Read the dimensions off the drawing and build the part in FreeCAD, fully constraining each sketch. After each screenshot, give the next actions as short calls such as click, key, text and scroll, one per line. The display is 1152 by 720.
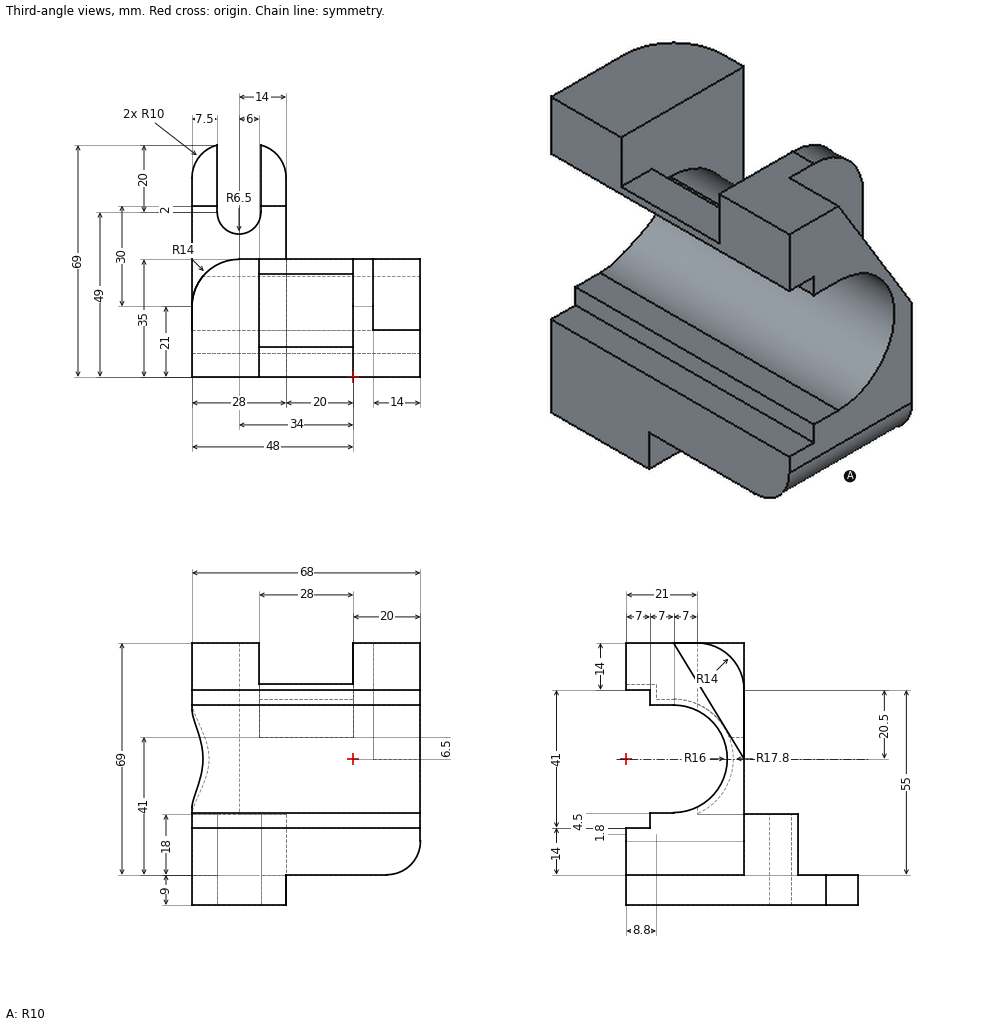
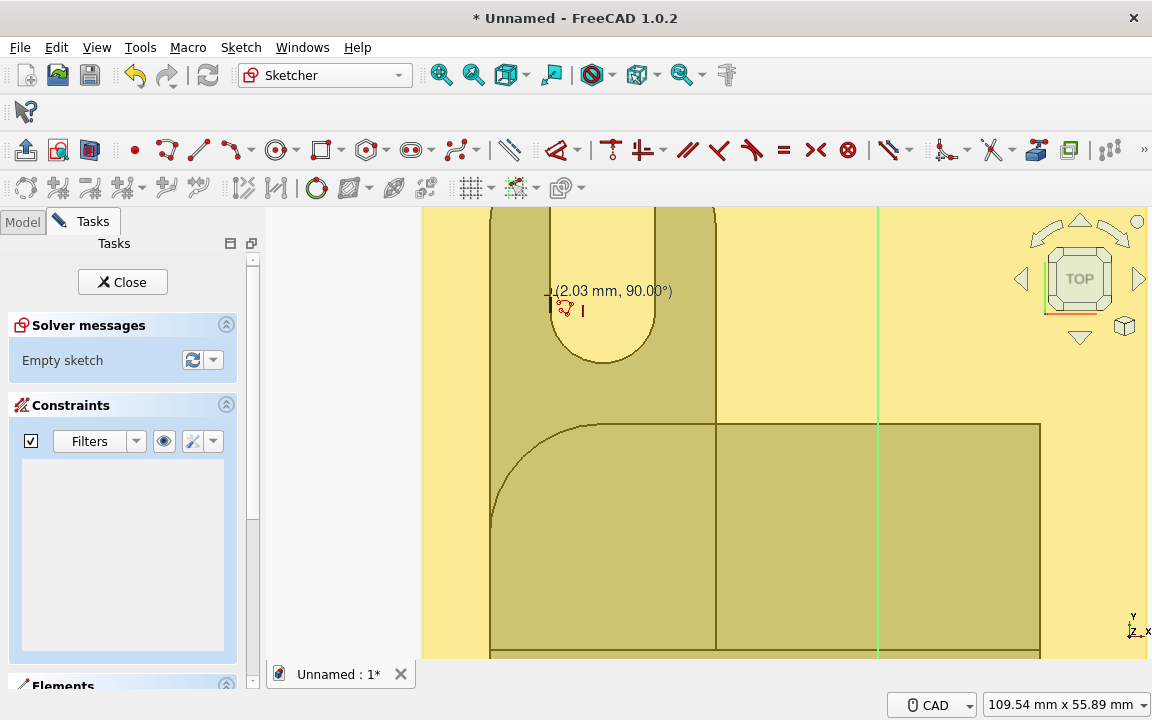
click(551, 295)
click(490, 295)
click(490, 537)
right_click(490, 537)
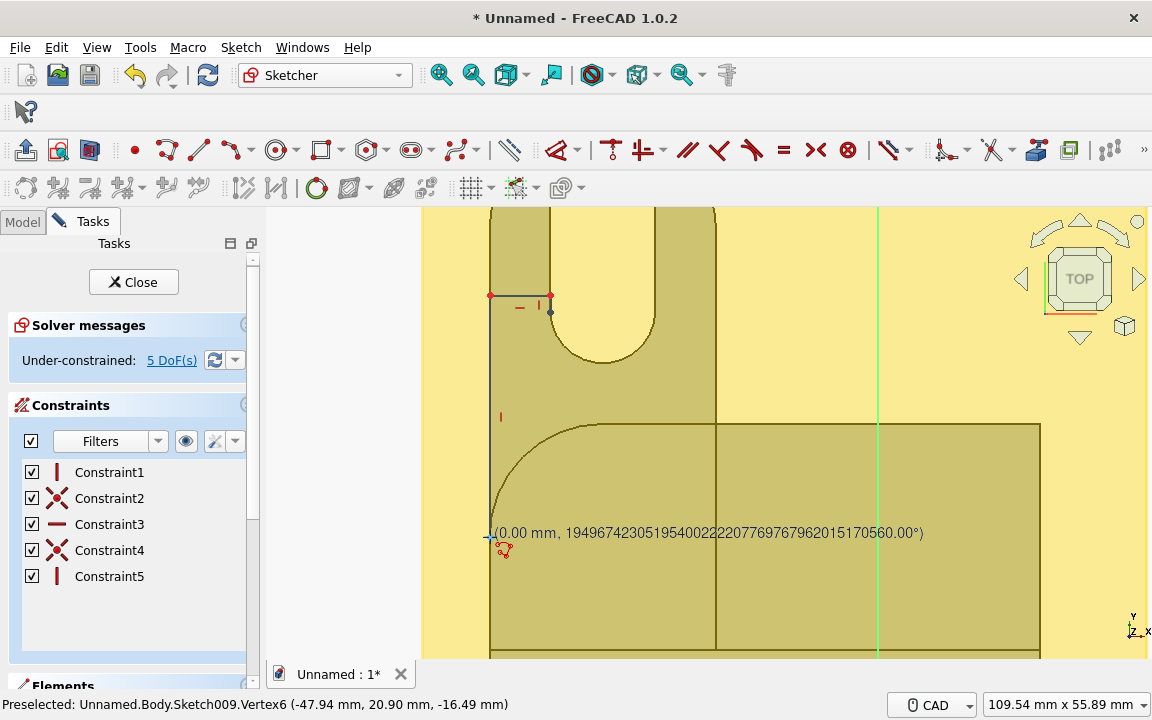
click(603, 424)
click(716, 424)
click(716, 295)
click(655, 295)
click(655, 311)
right_click(655, 311)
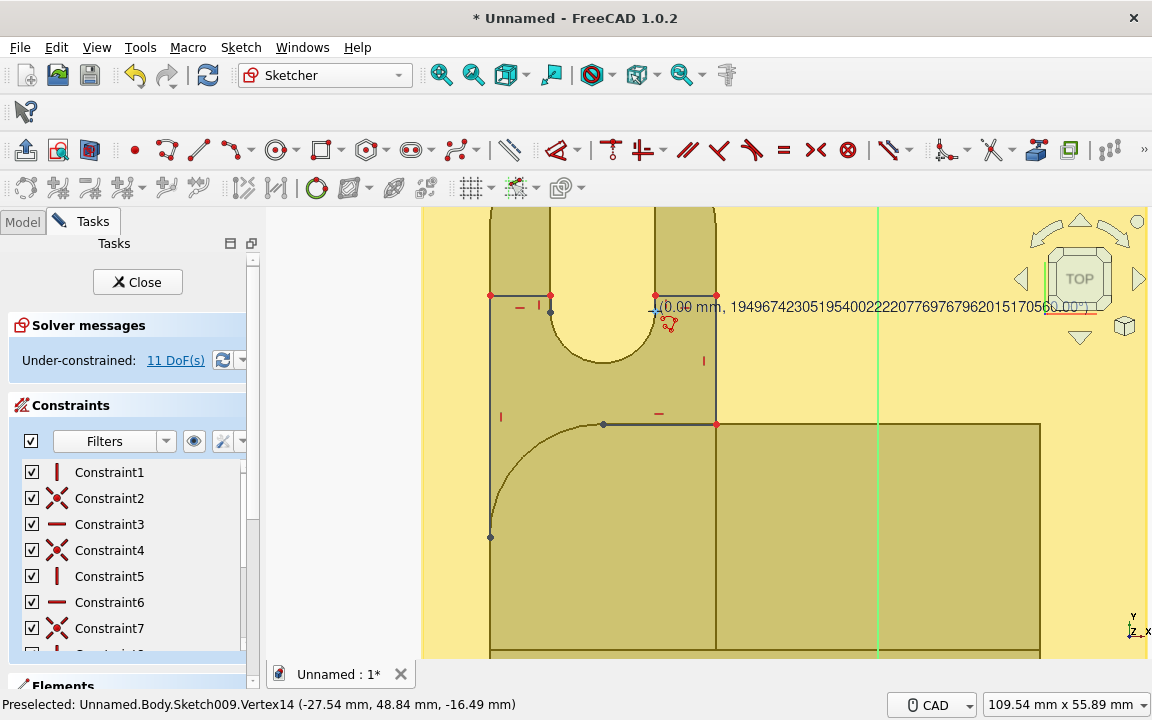
key(g)
key(3)
key(a)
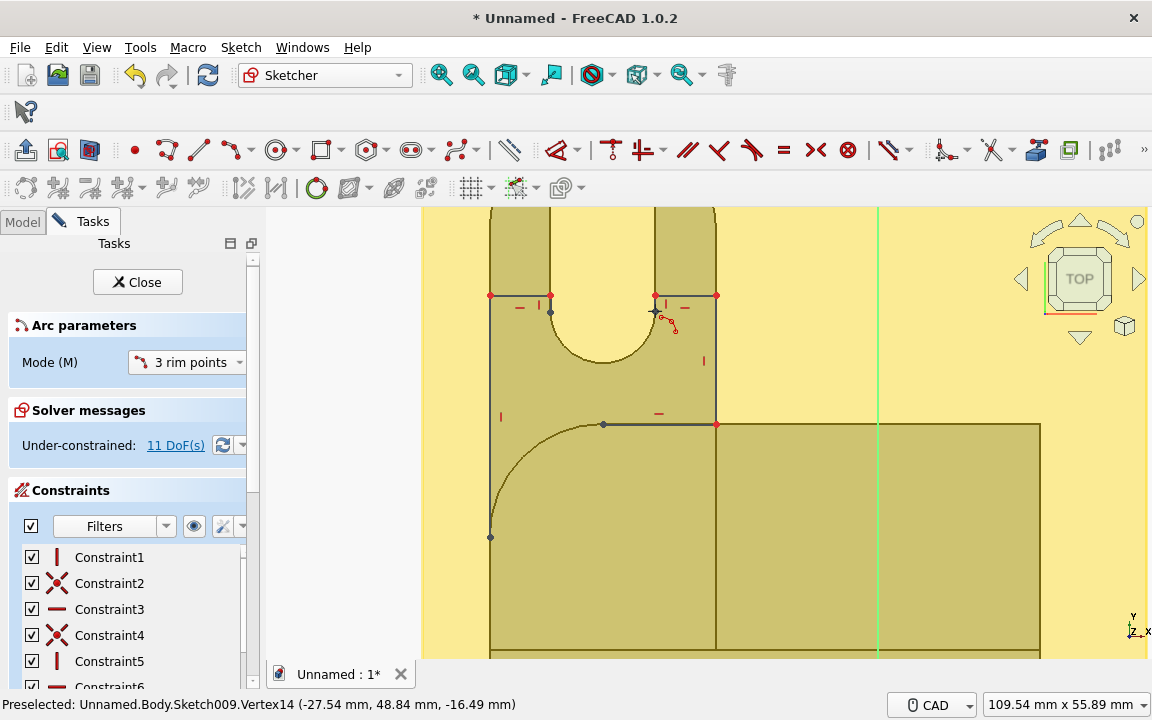
click(490, 538)
click(603, 425)
click(523, 457)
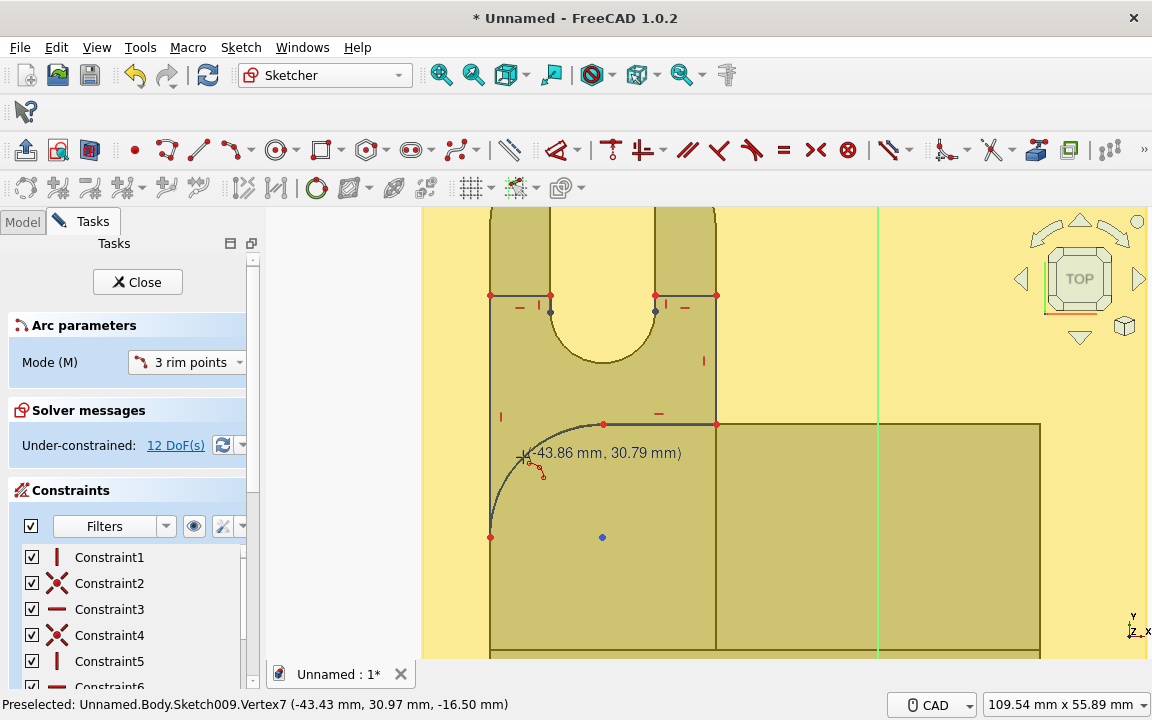
scroll(655, 311, up, 4)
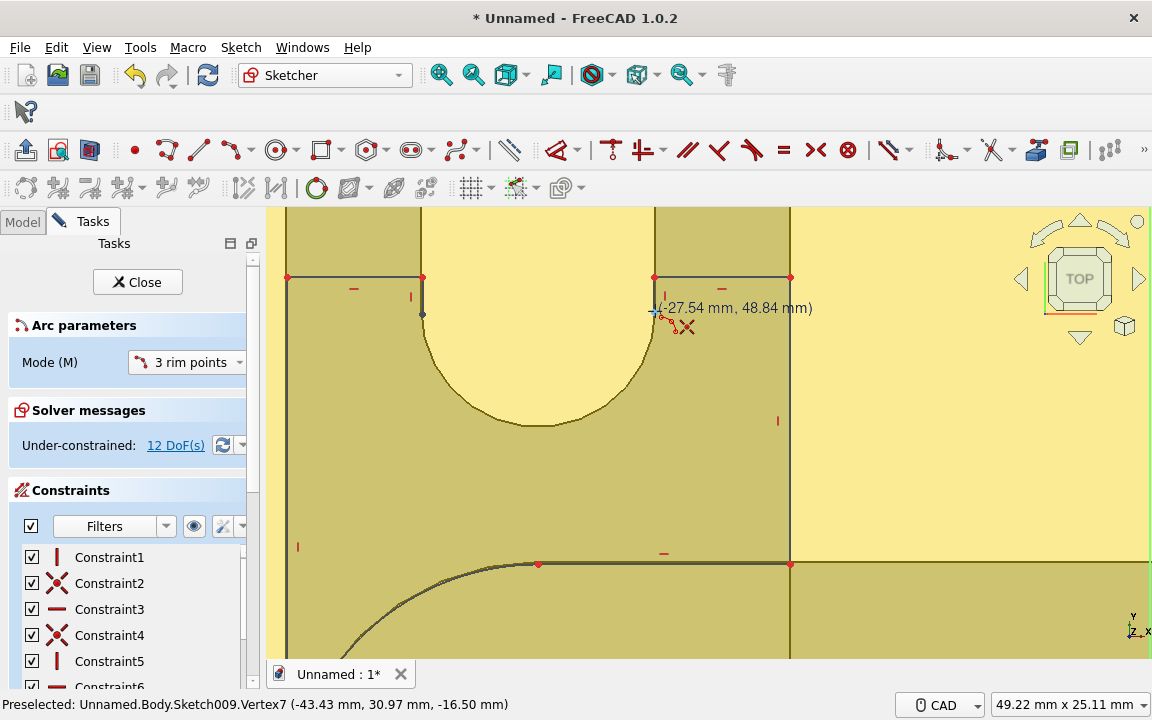
click(654, 313)
click(423, 315)
click(538, 427)
key(Escape)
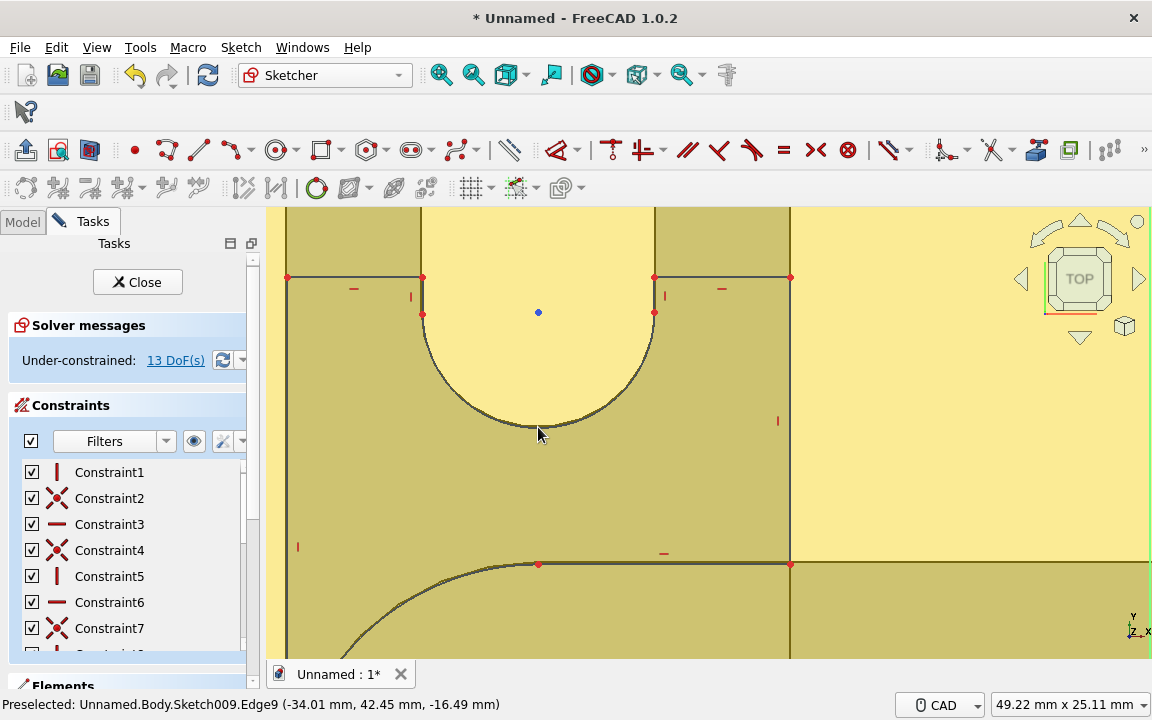
scroll(423, 304, up, 2)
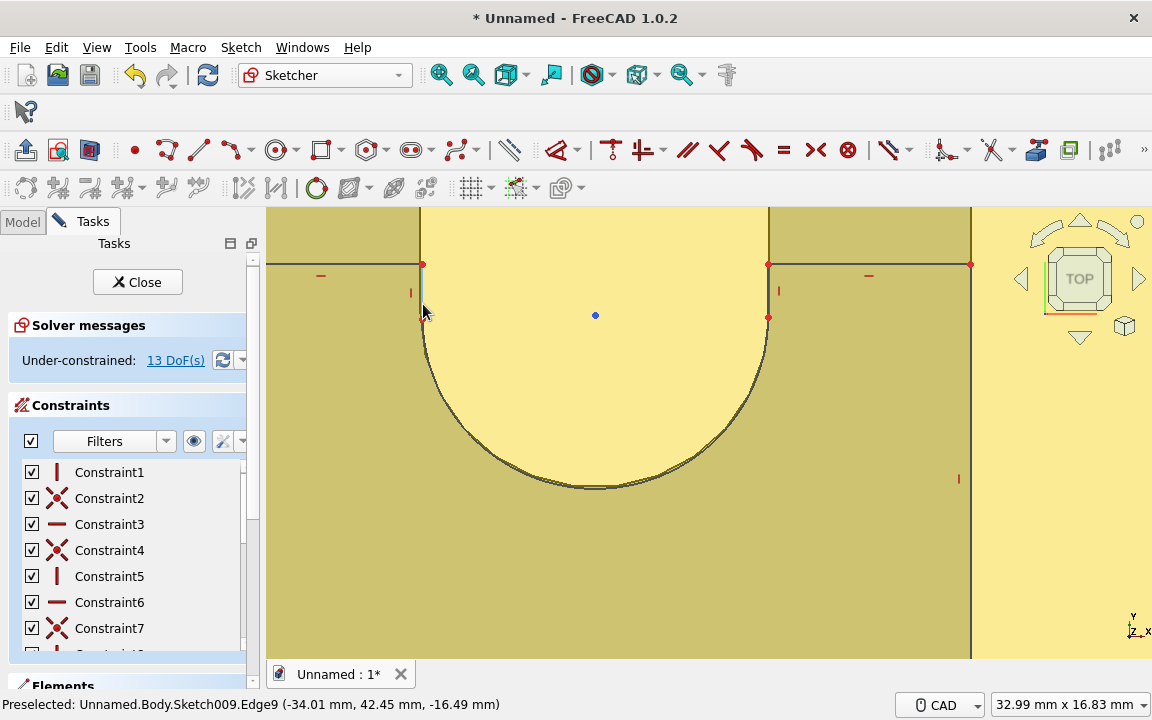
click(422, 303)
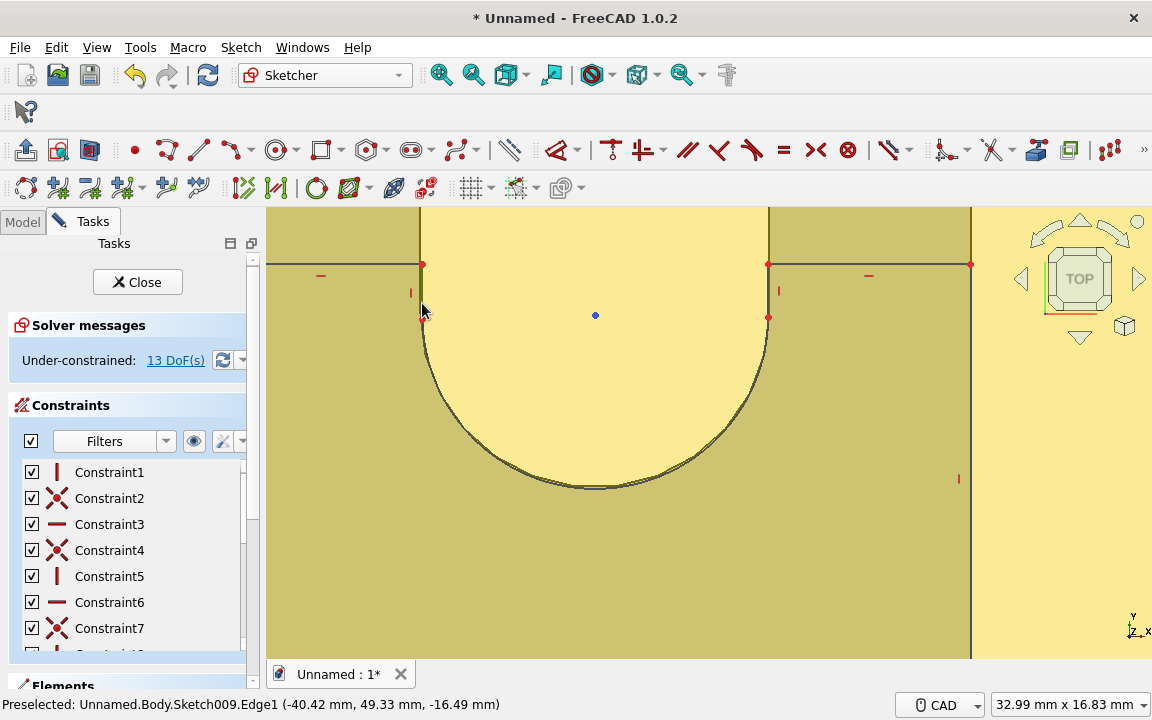
scroll(584, 304, down, 8)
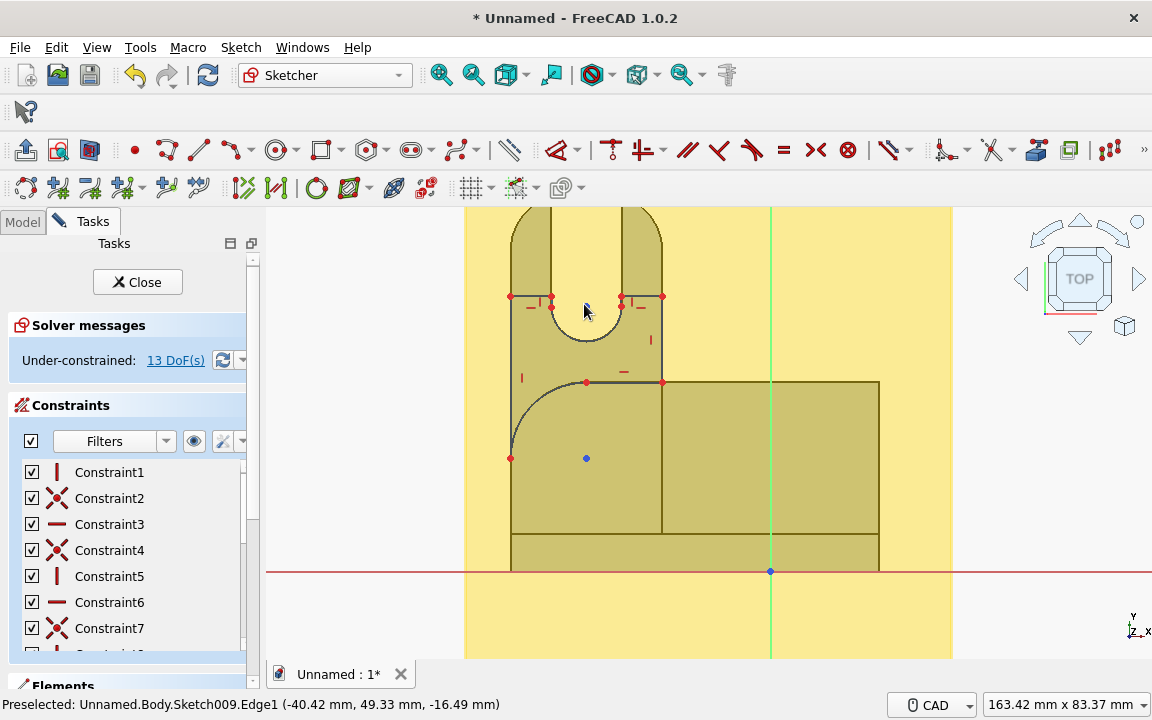
click(566, 335)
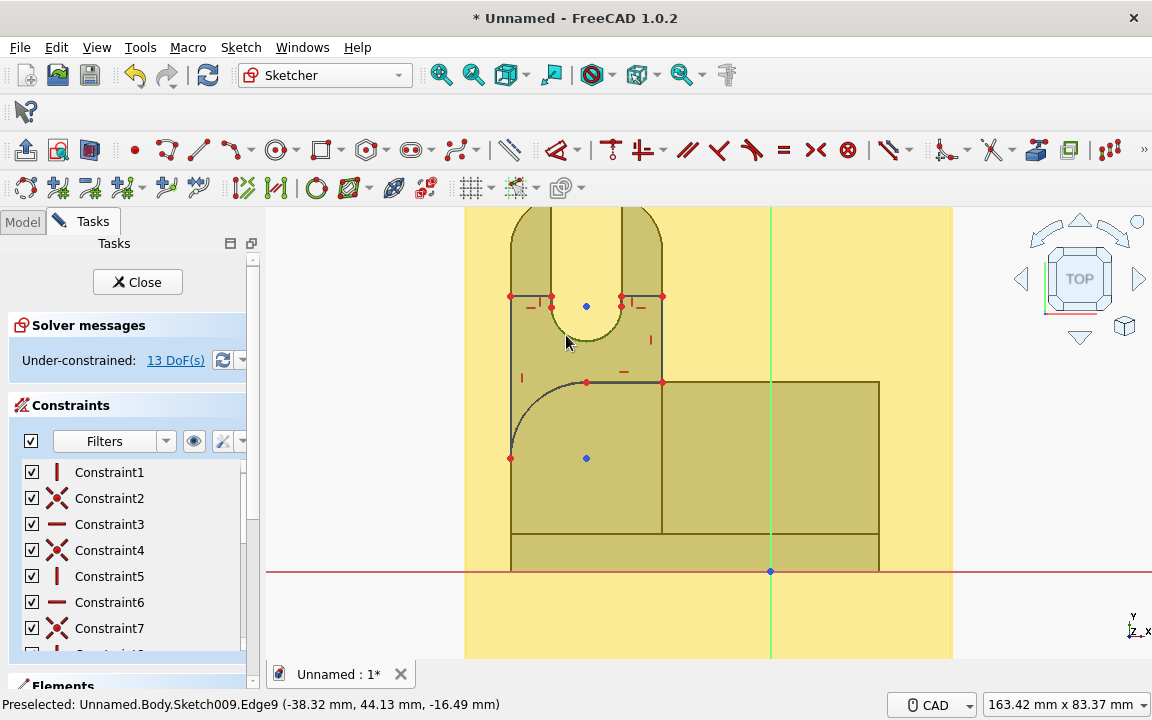
click(752, 150)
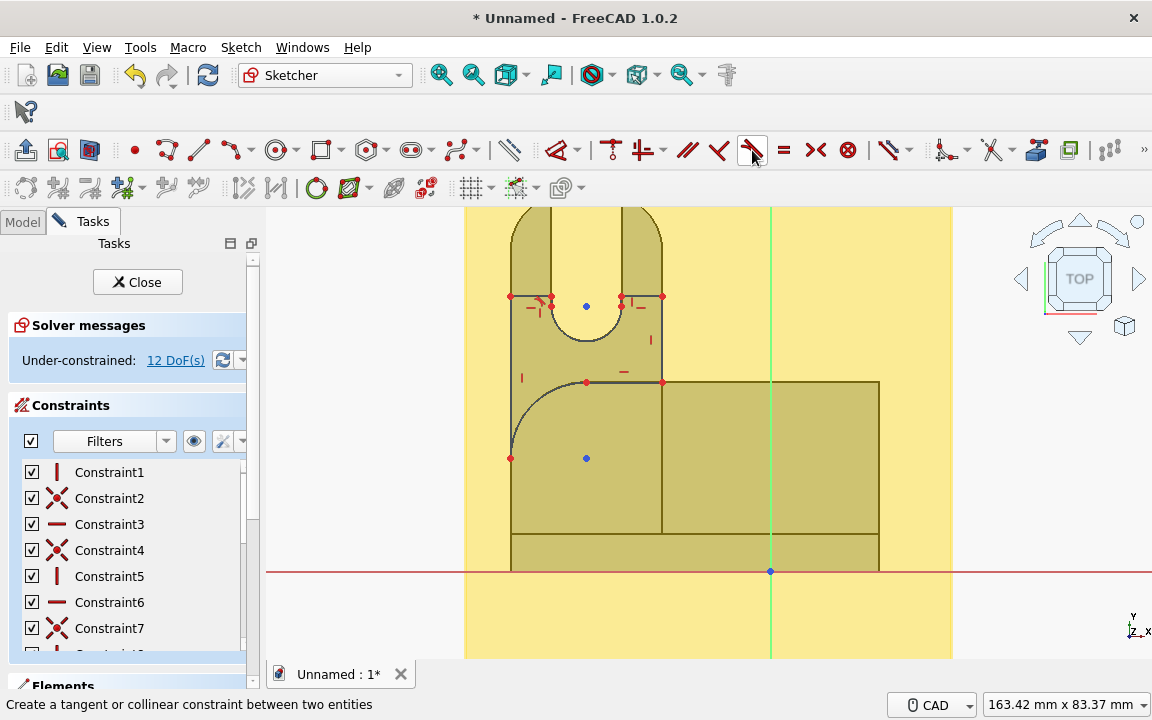
click(511, 345)